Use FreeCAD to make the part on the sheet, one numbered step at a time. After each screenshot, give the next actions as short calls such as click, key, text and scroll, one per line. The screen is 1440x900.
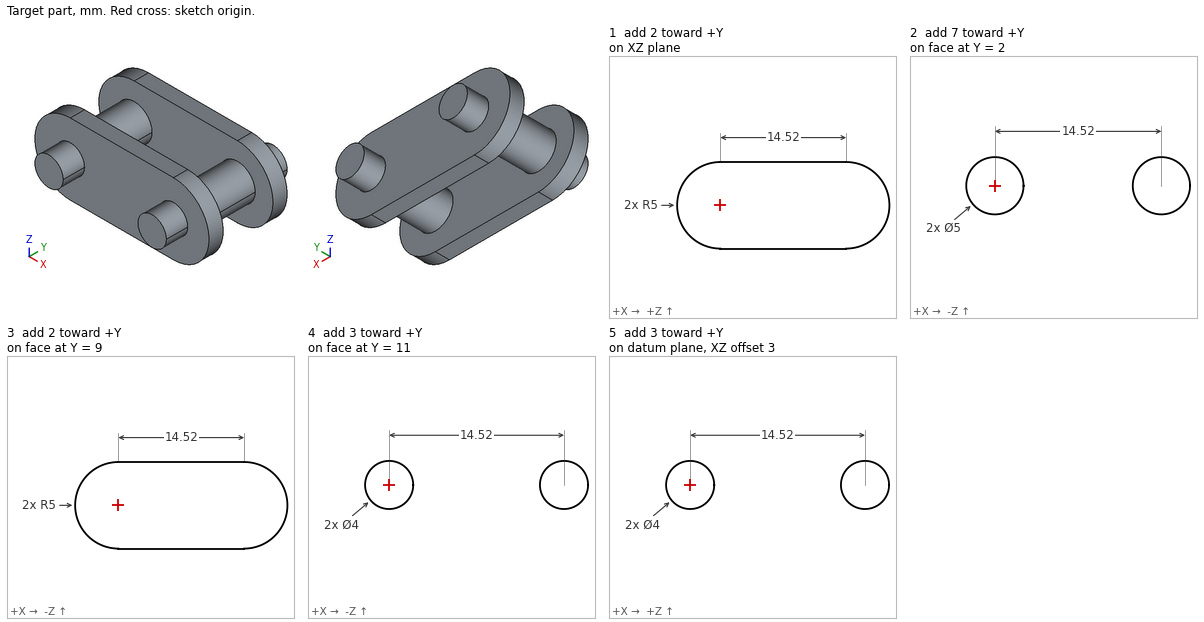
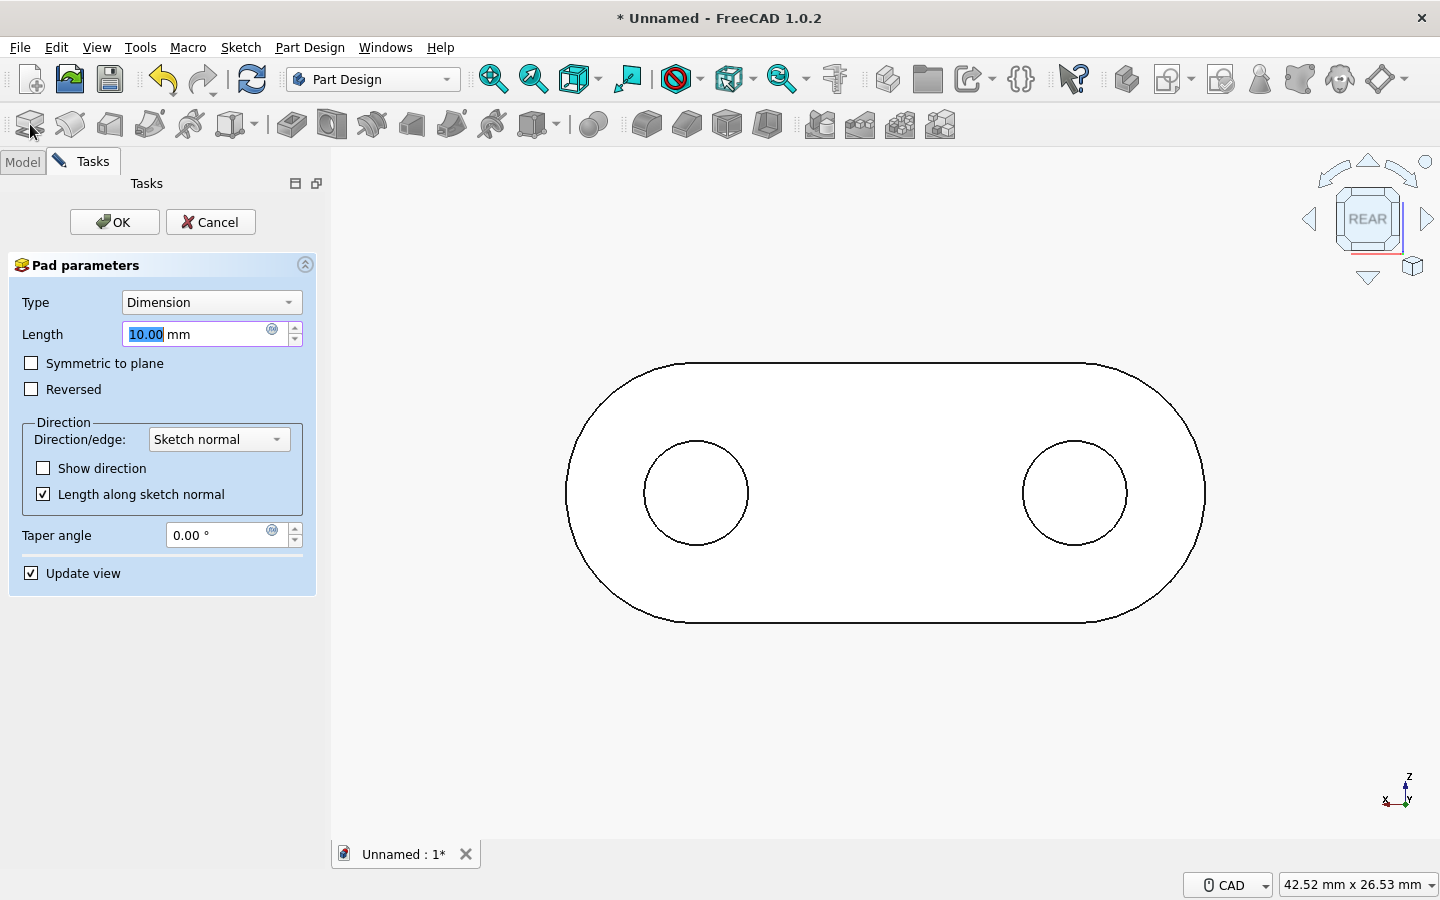
text(3)
key(Tab)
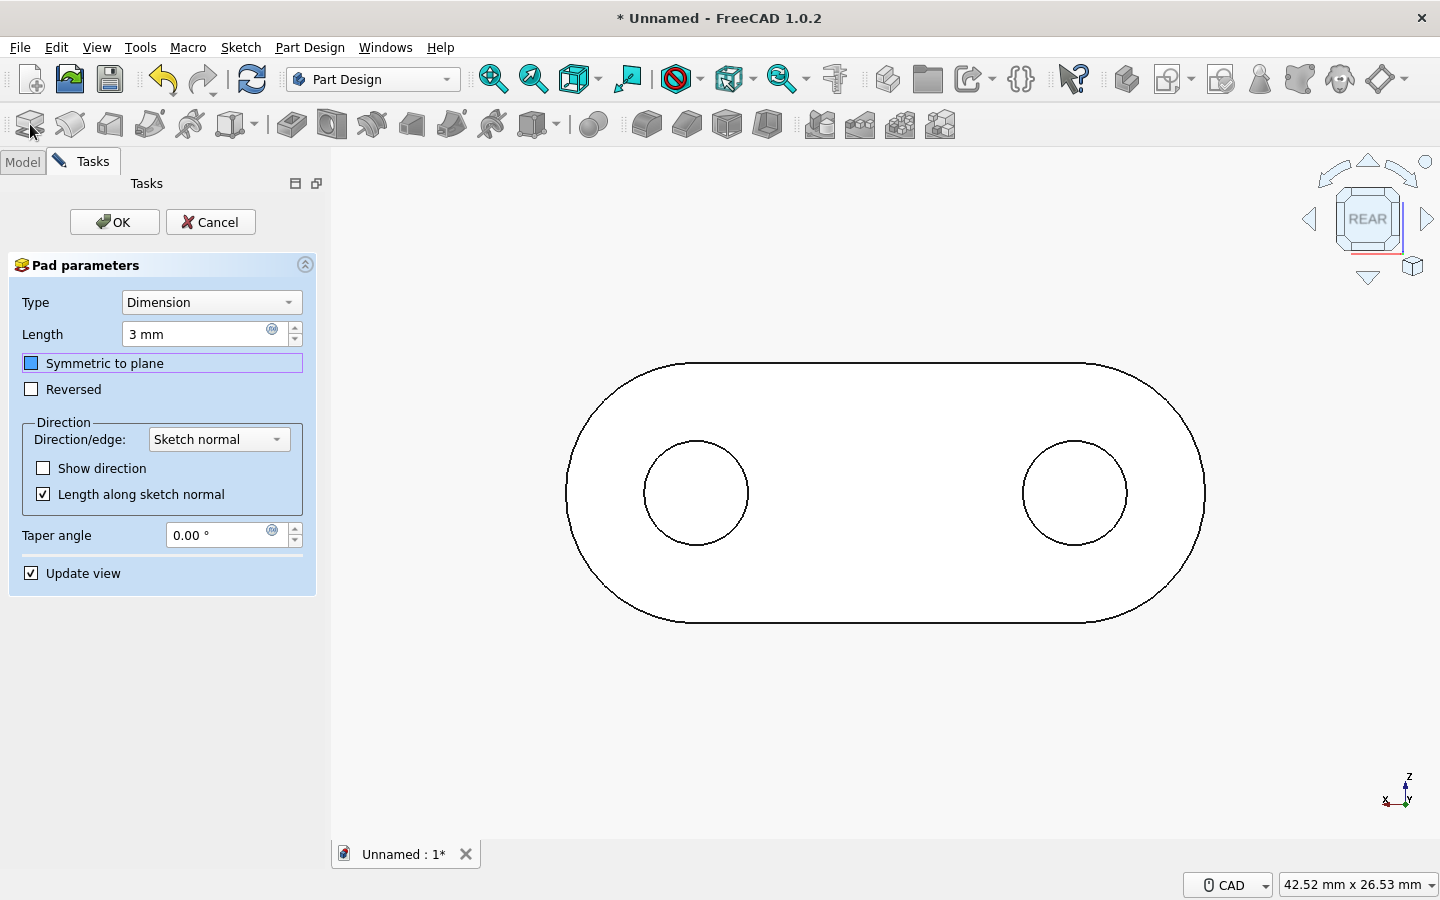
click(115, 222)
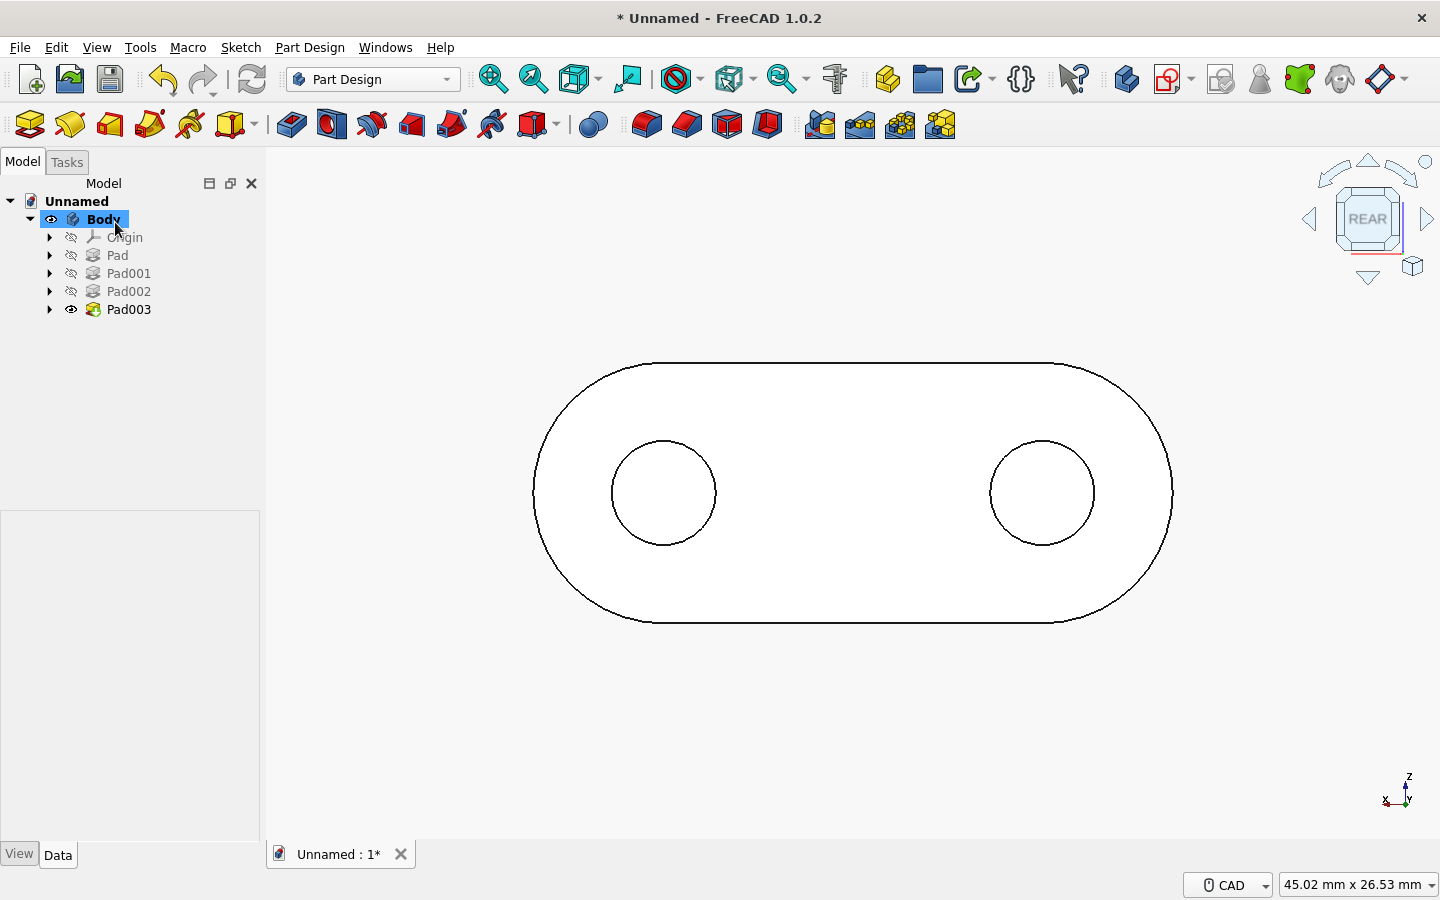
click(50, 237)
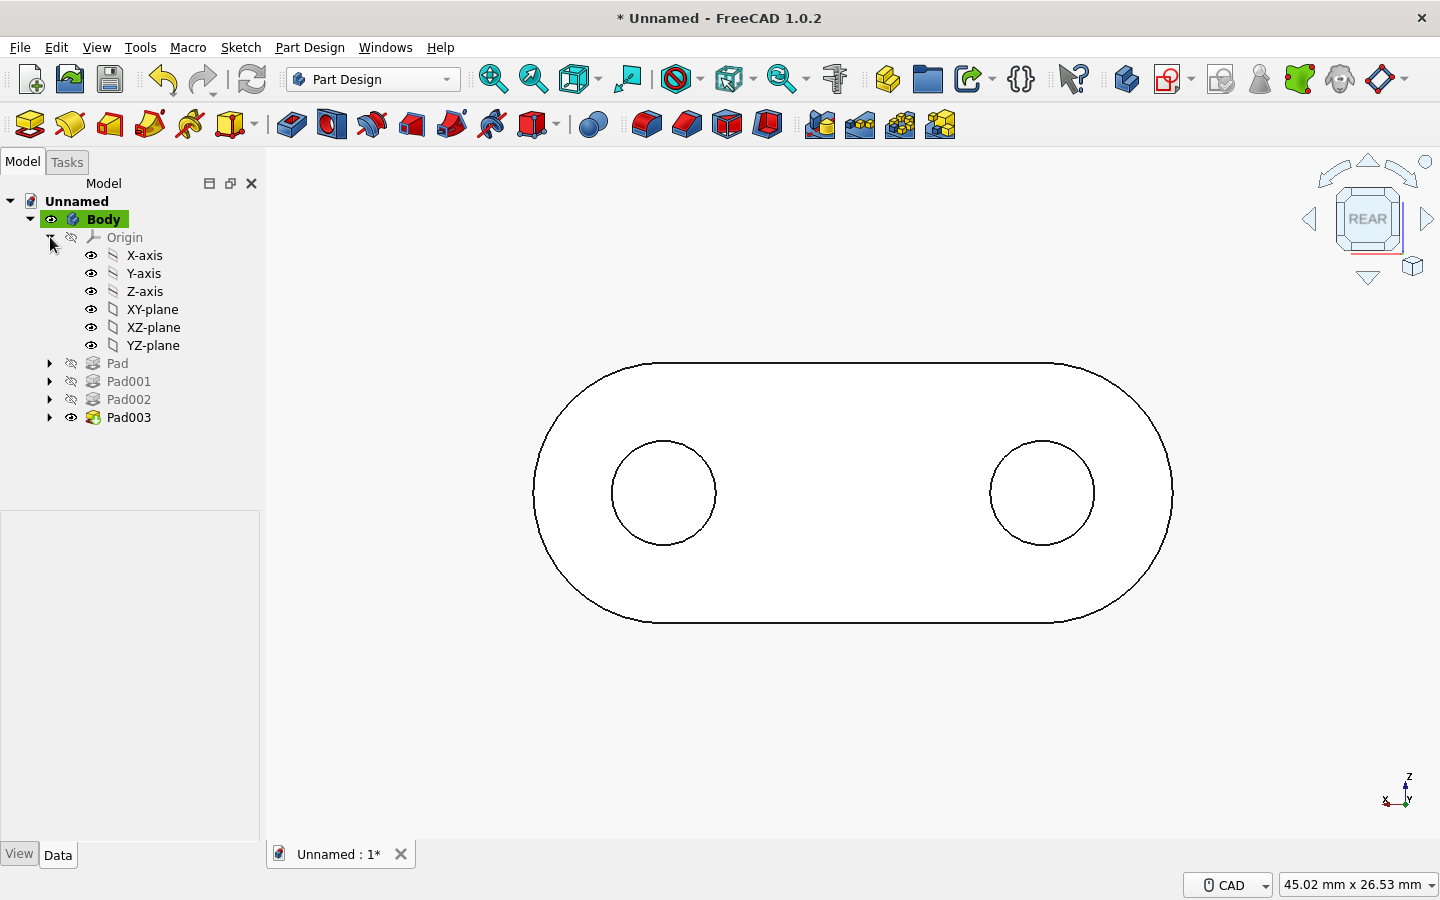
click(136, 327)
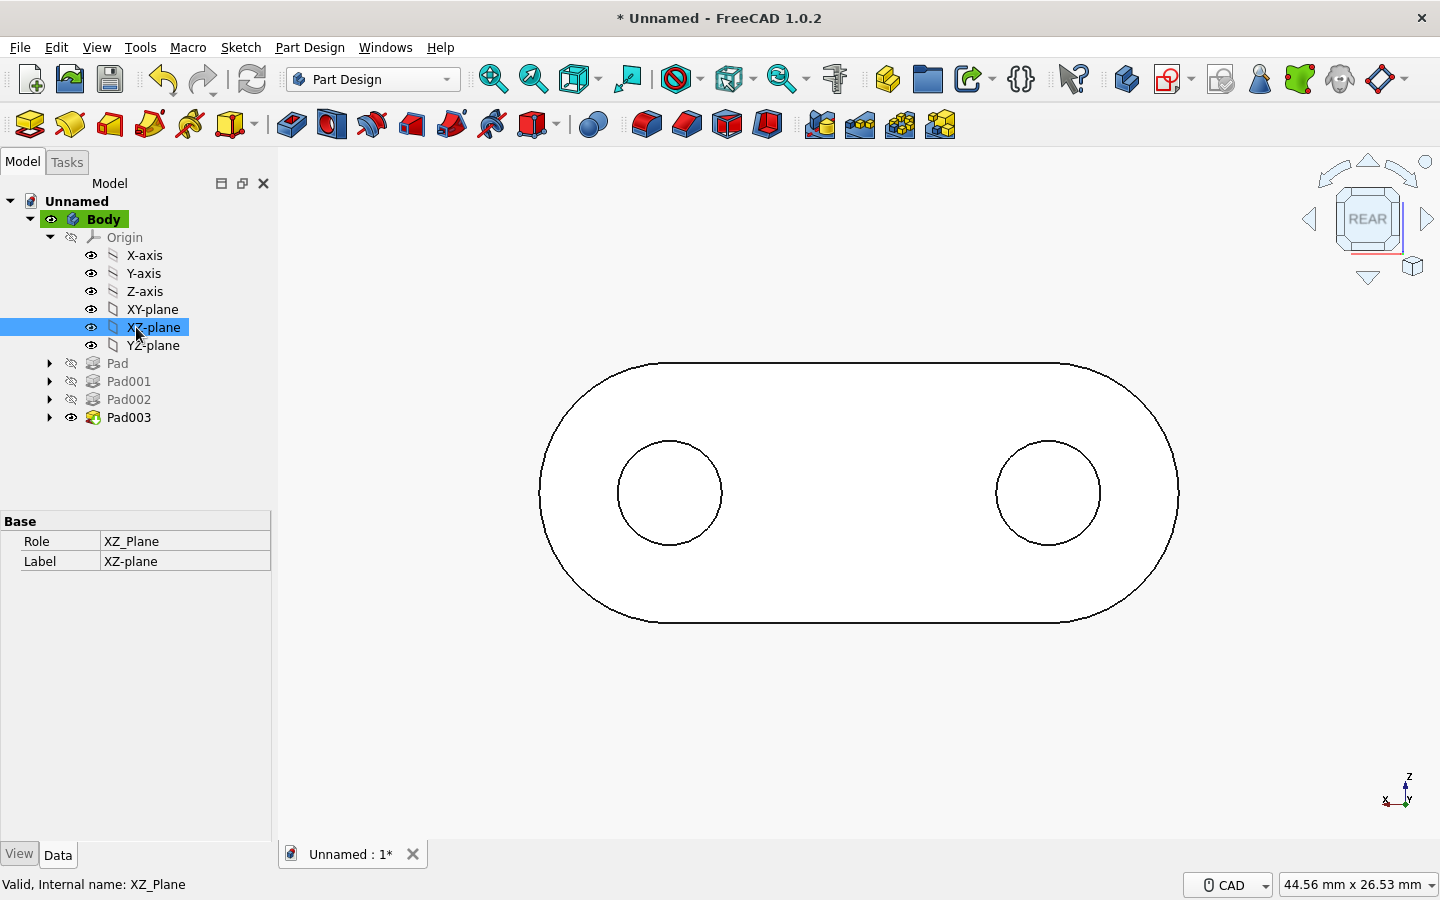
click(1380, 80)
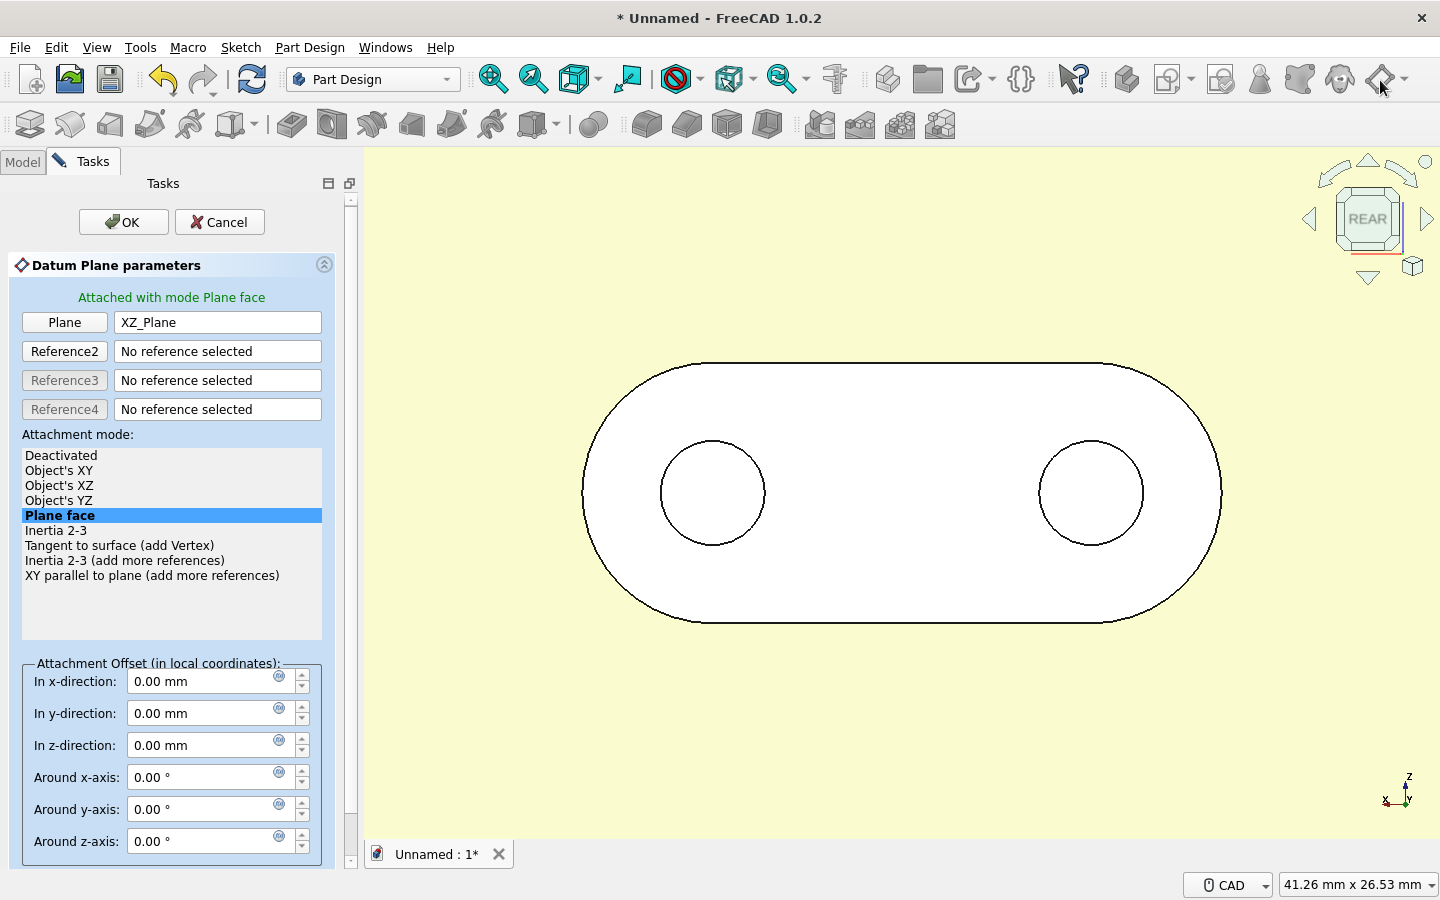
triple_click(210, 745)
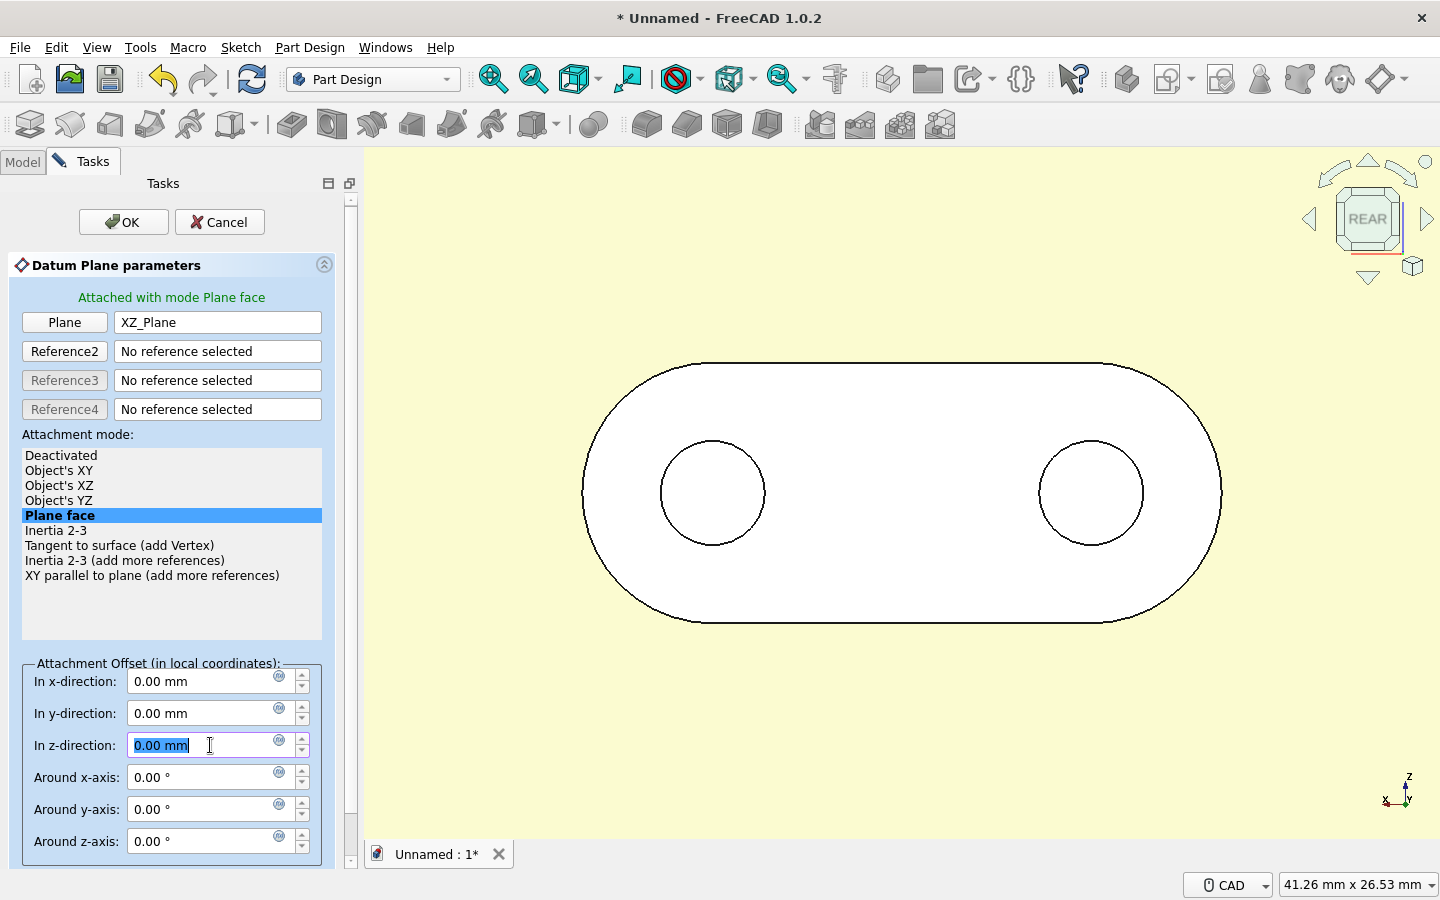
text(3)
key(Tab)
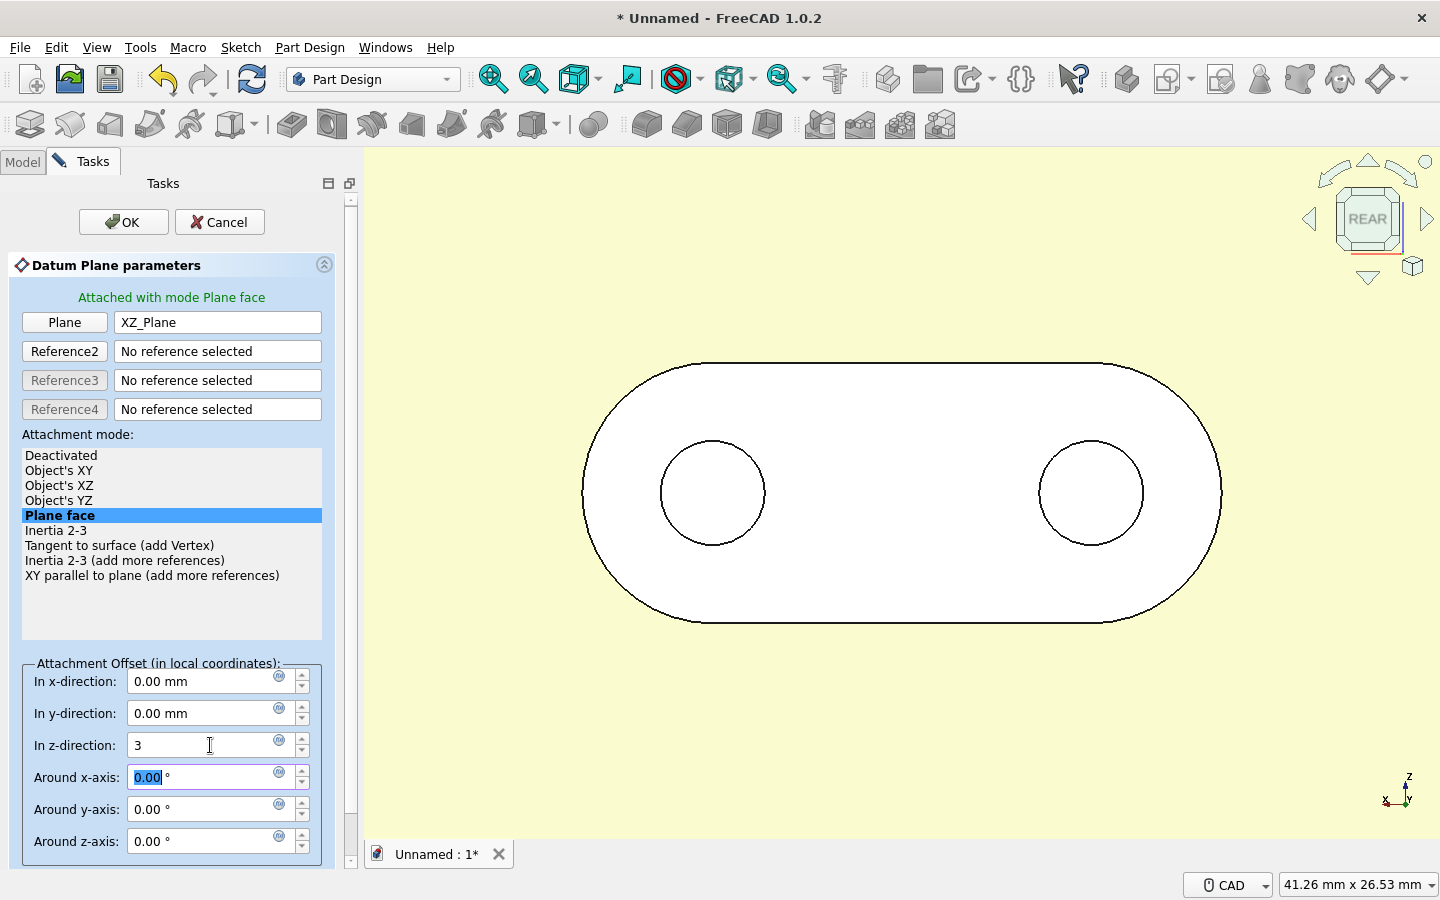
click(124, 222)